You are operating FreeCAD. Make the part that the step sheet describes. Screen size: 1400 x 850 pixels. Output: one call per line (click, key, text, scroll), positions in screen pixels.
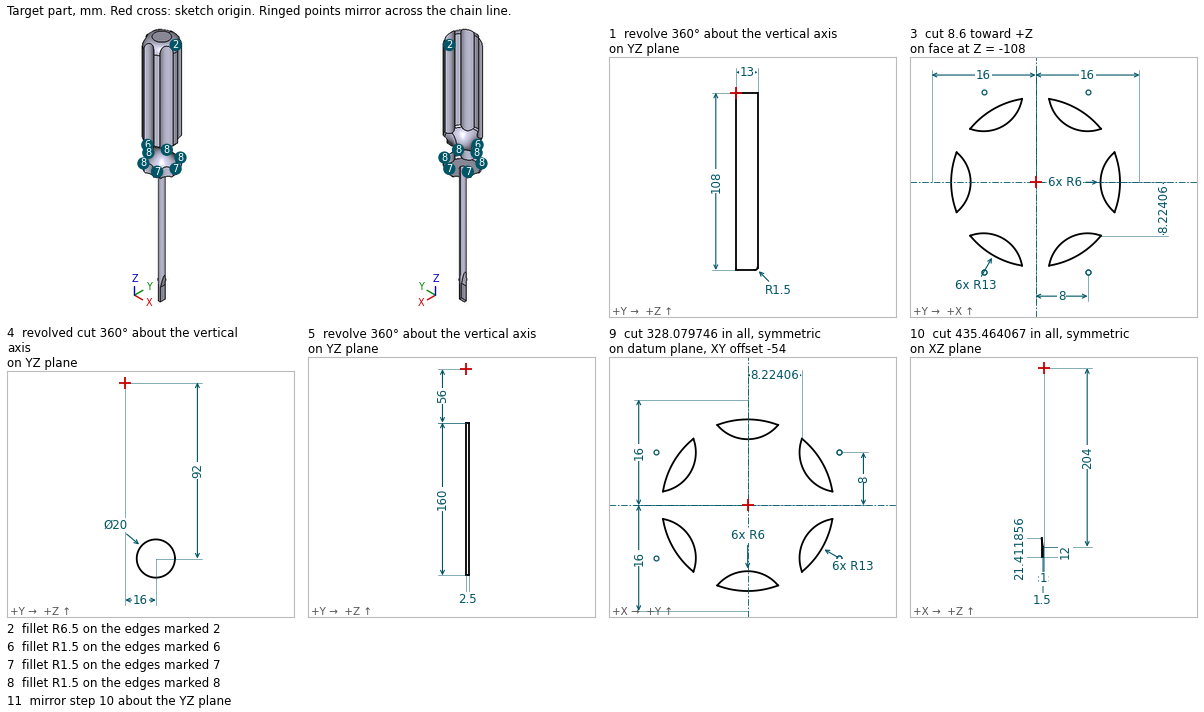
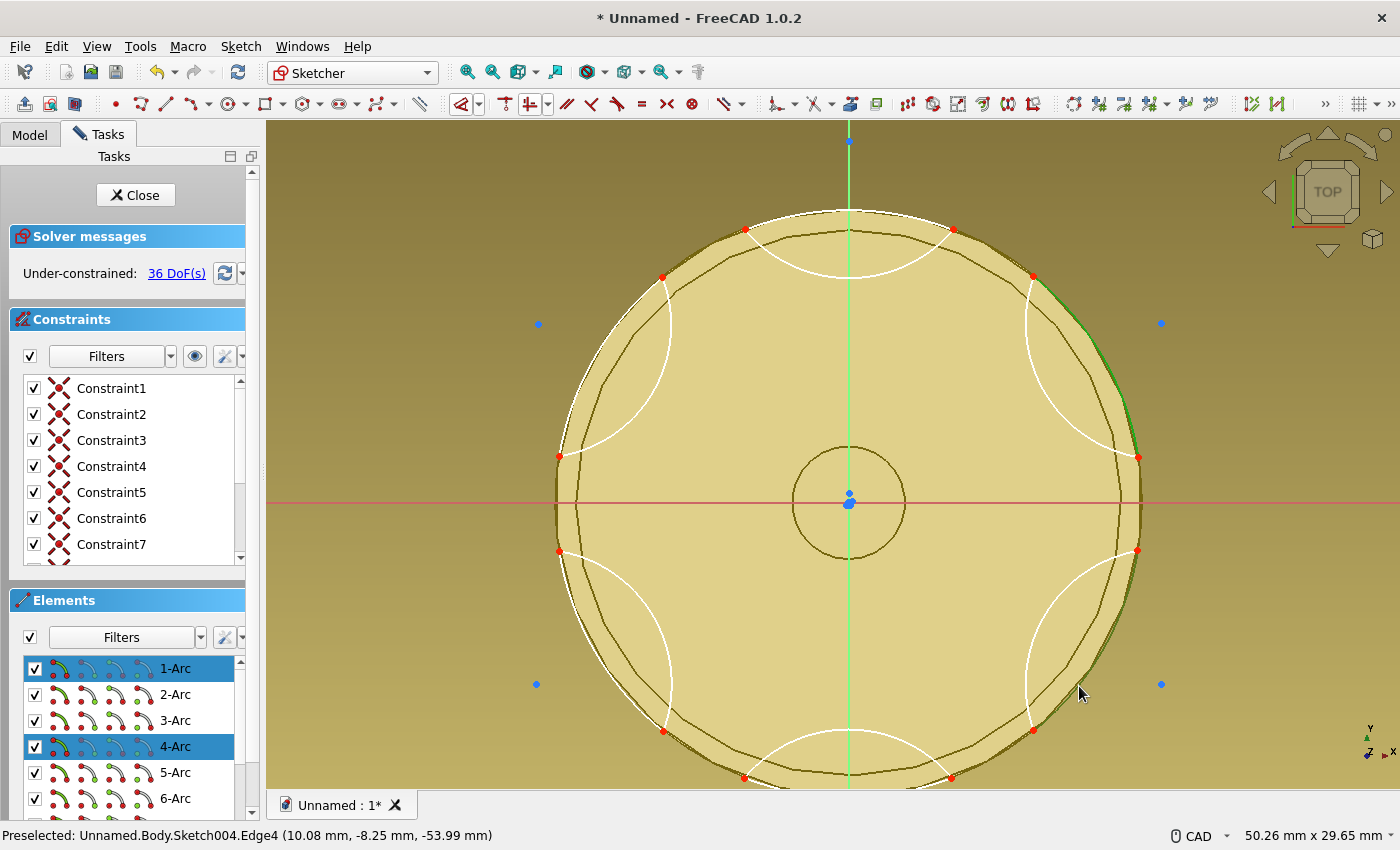
key(c)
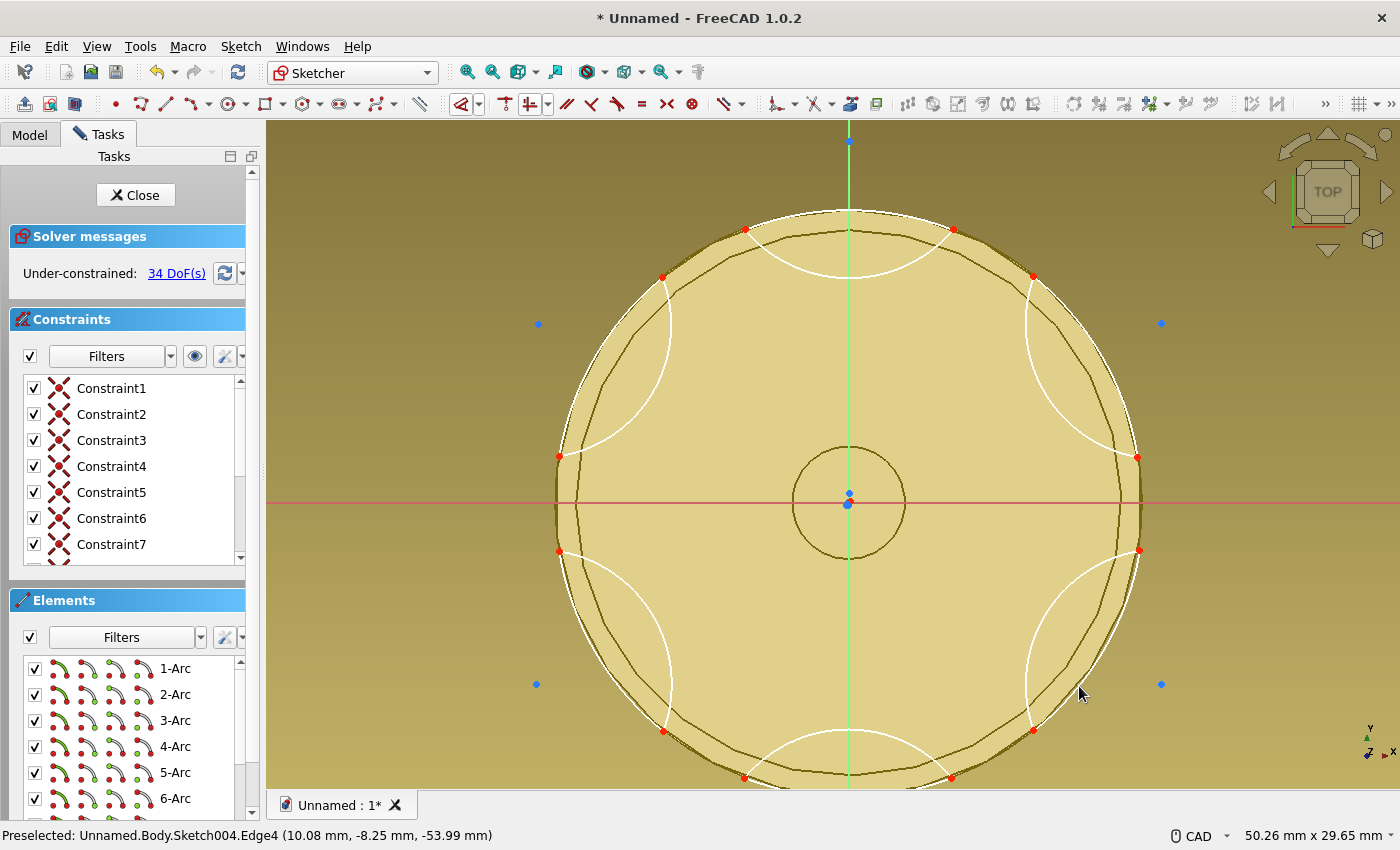
click(1121, 396)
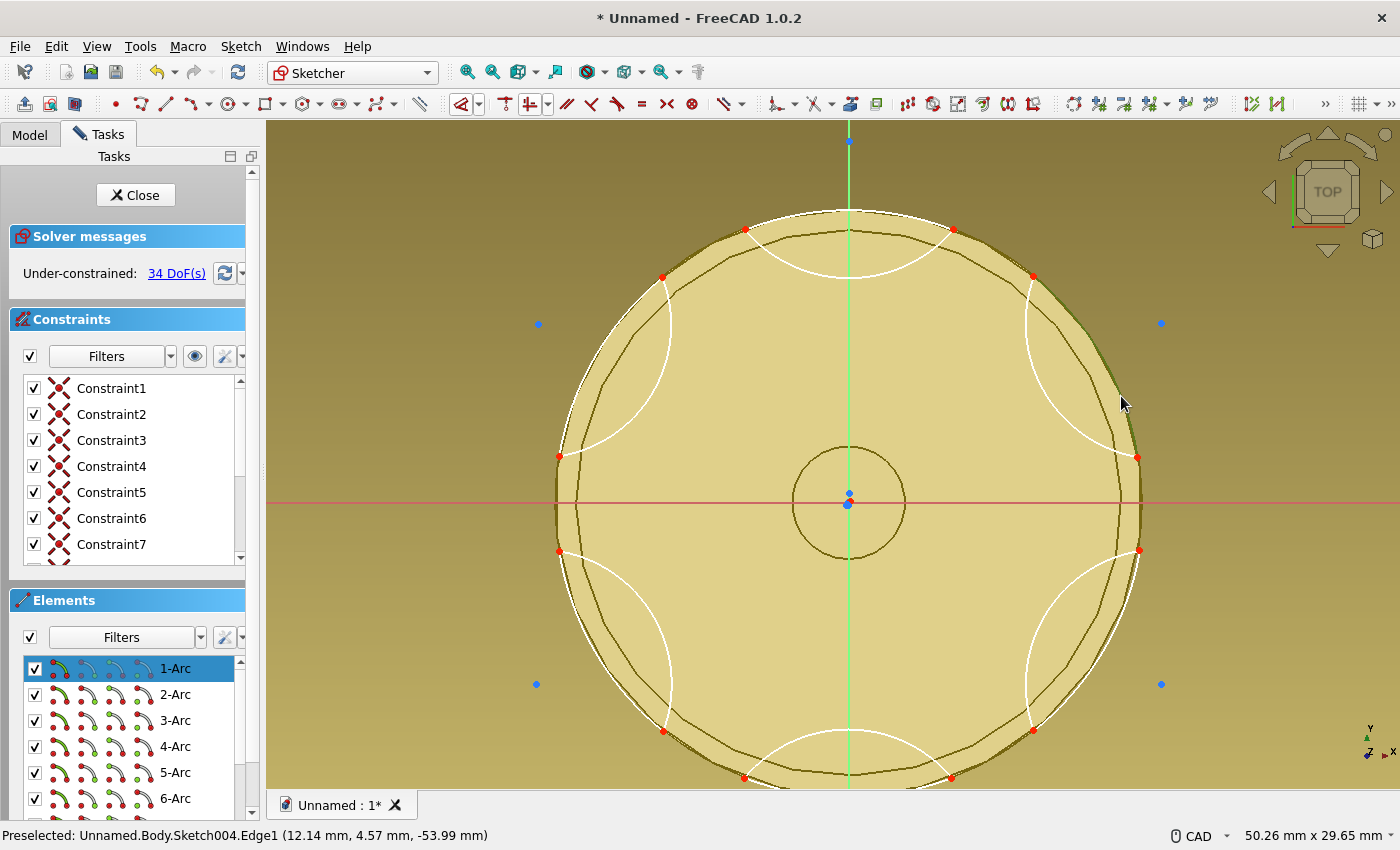
scroll(594, 356, down, 2)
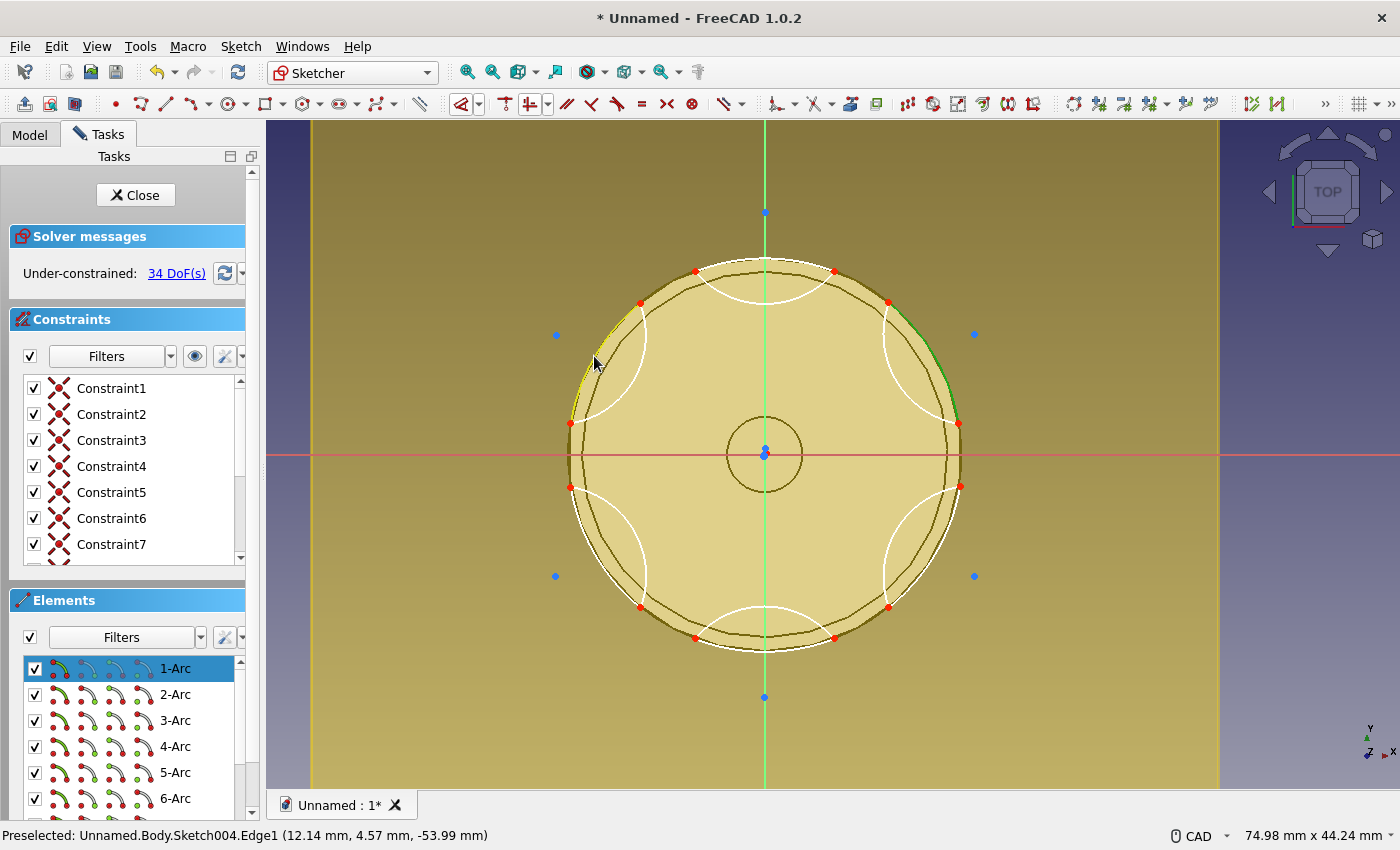
click(736, 650)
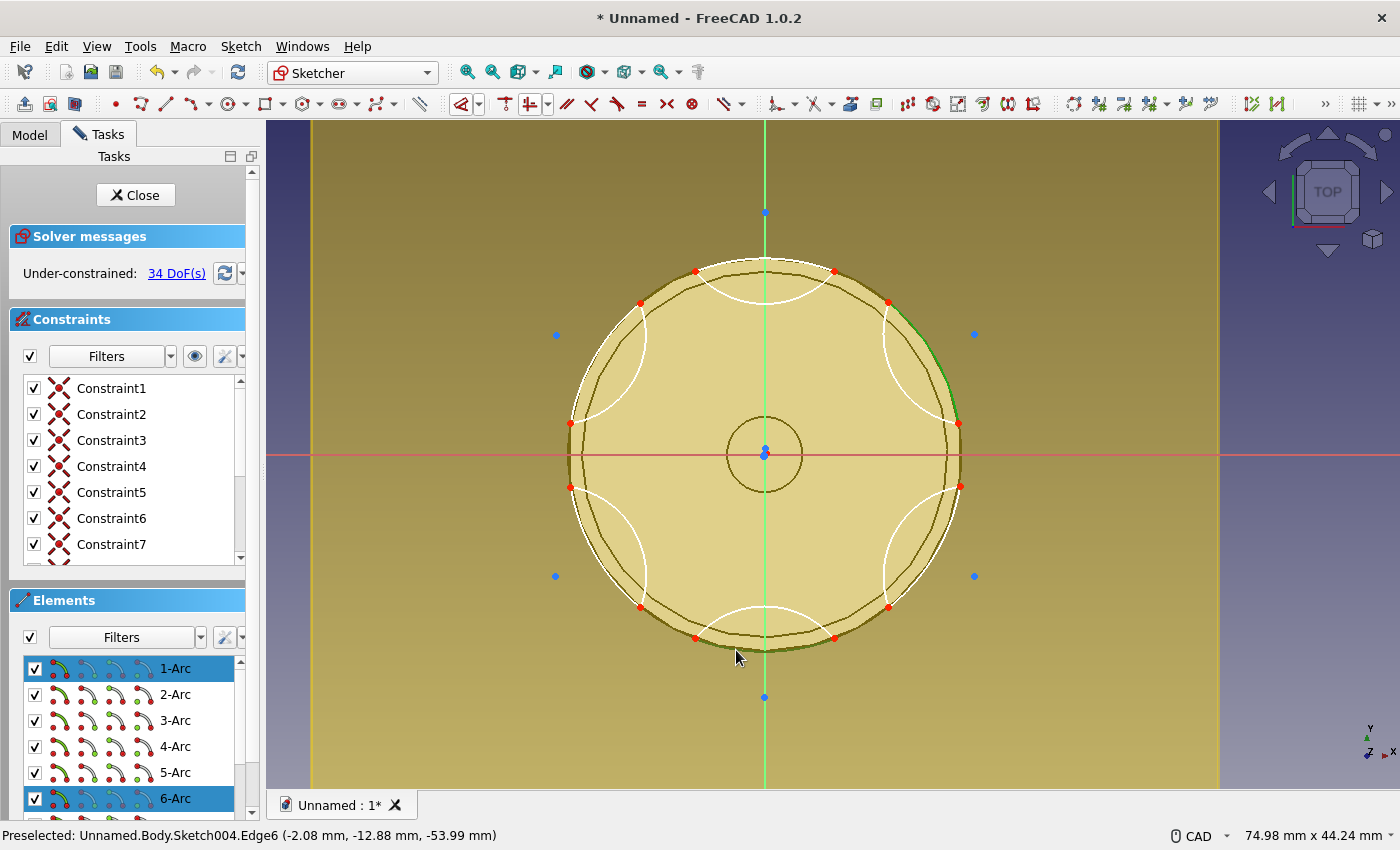
click(505, 104)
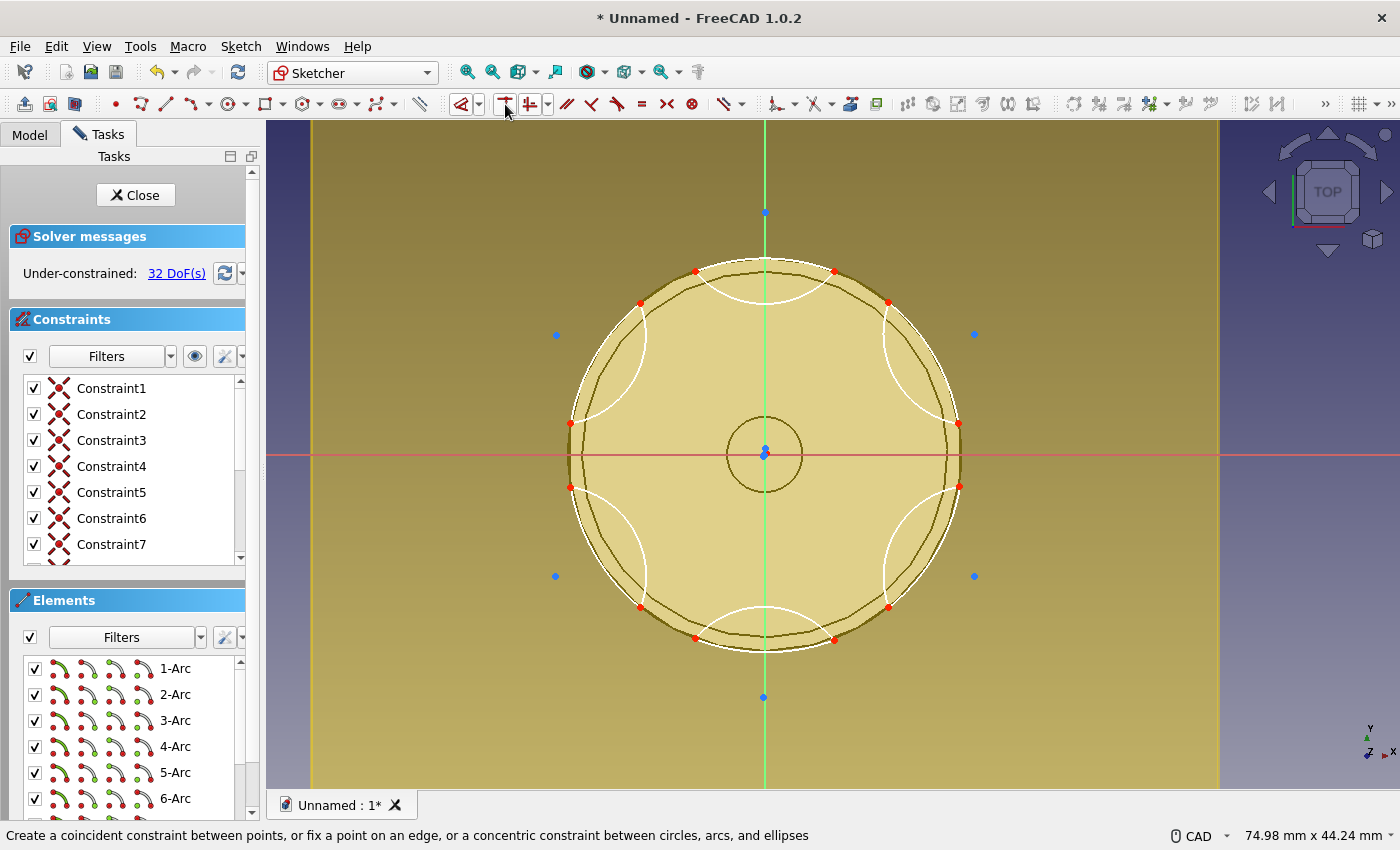
click(947, 383)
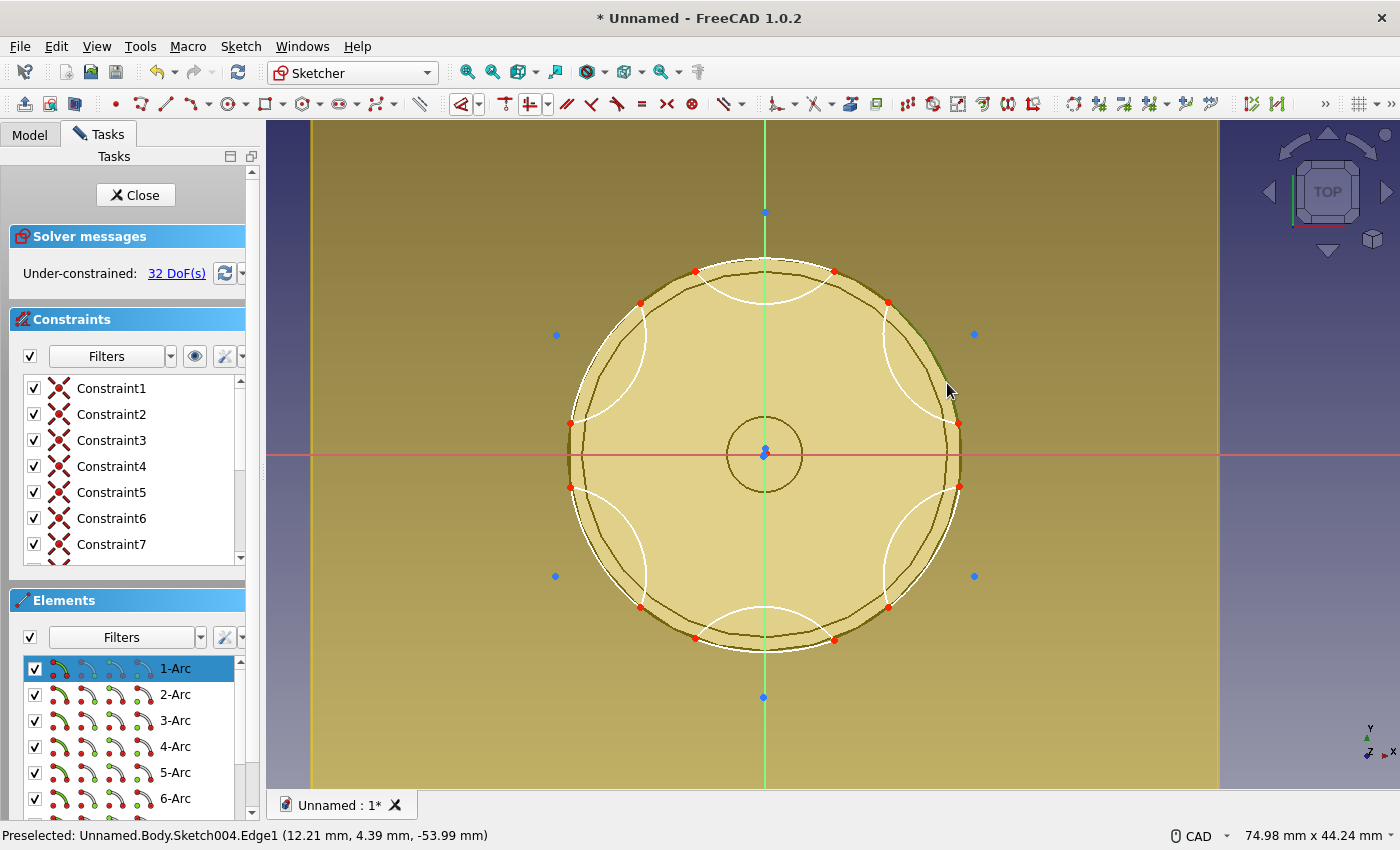
click(582, 528)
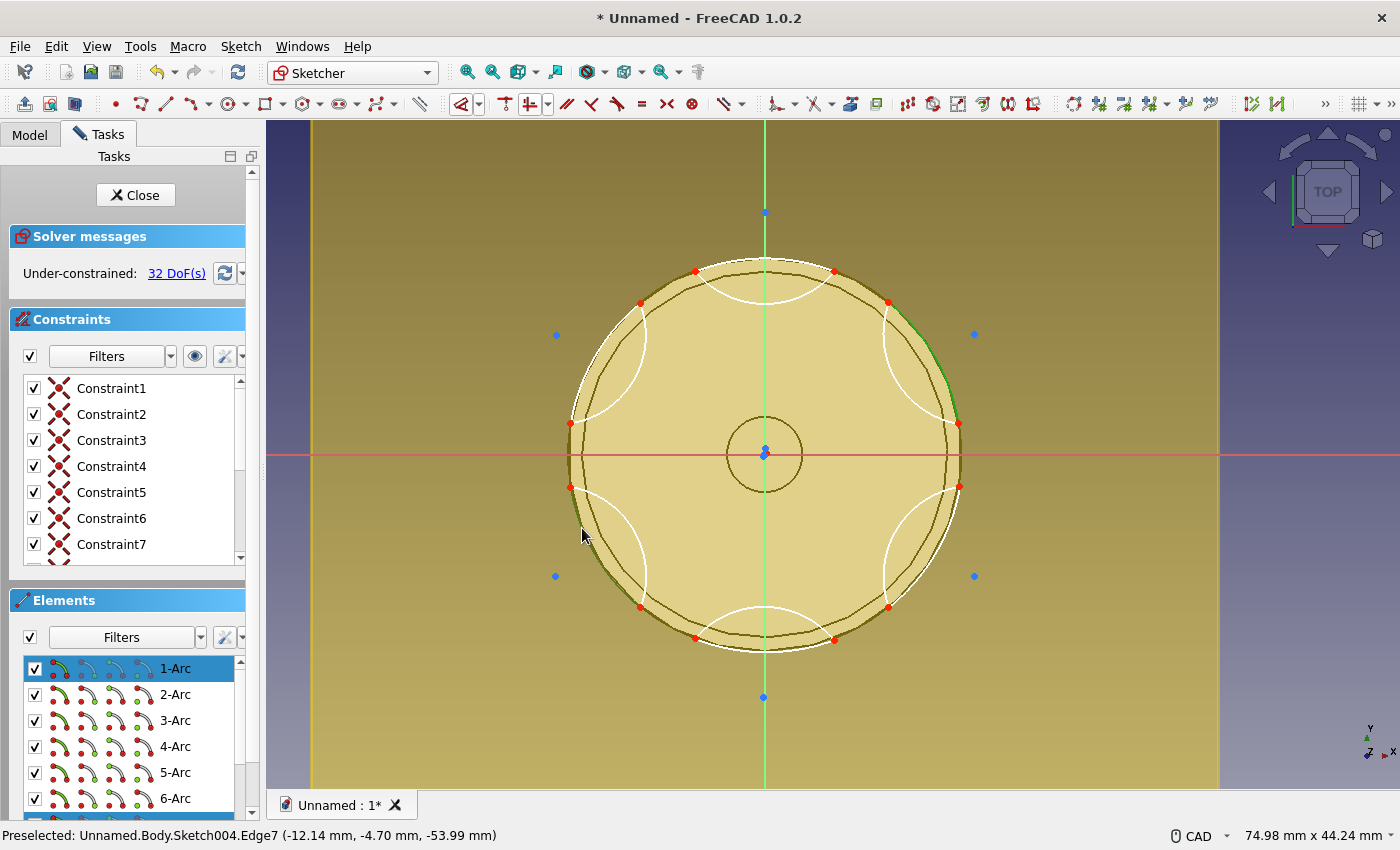
key(c)